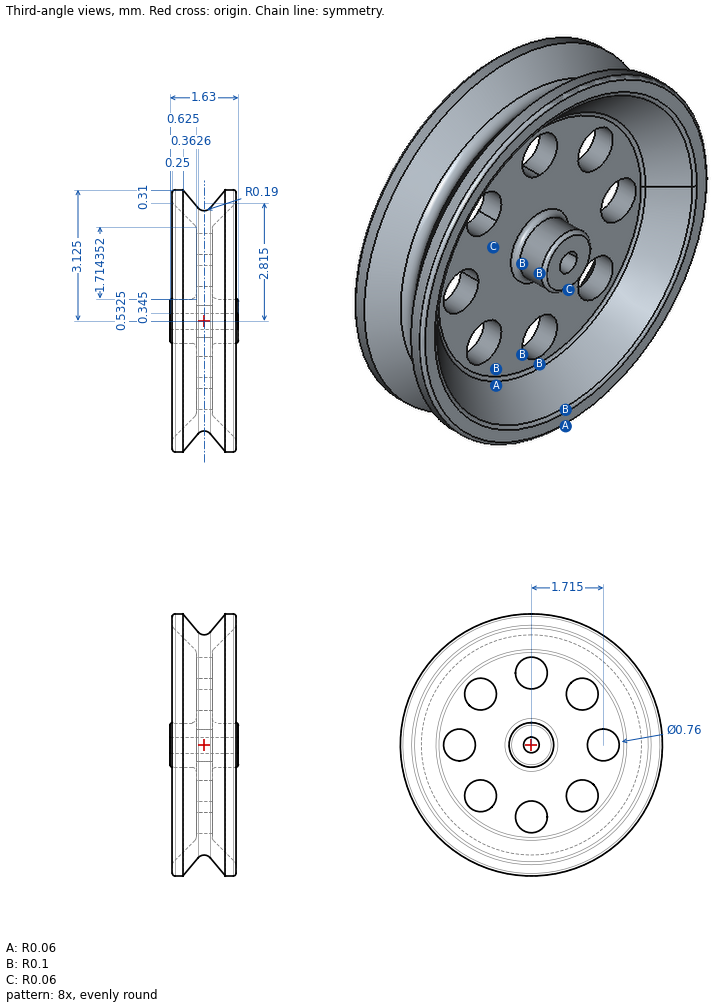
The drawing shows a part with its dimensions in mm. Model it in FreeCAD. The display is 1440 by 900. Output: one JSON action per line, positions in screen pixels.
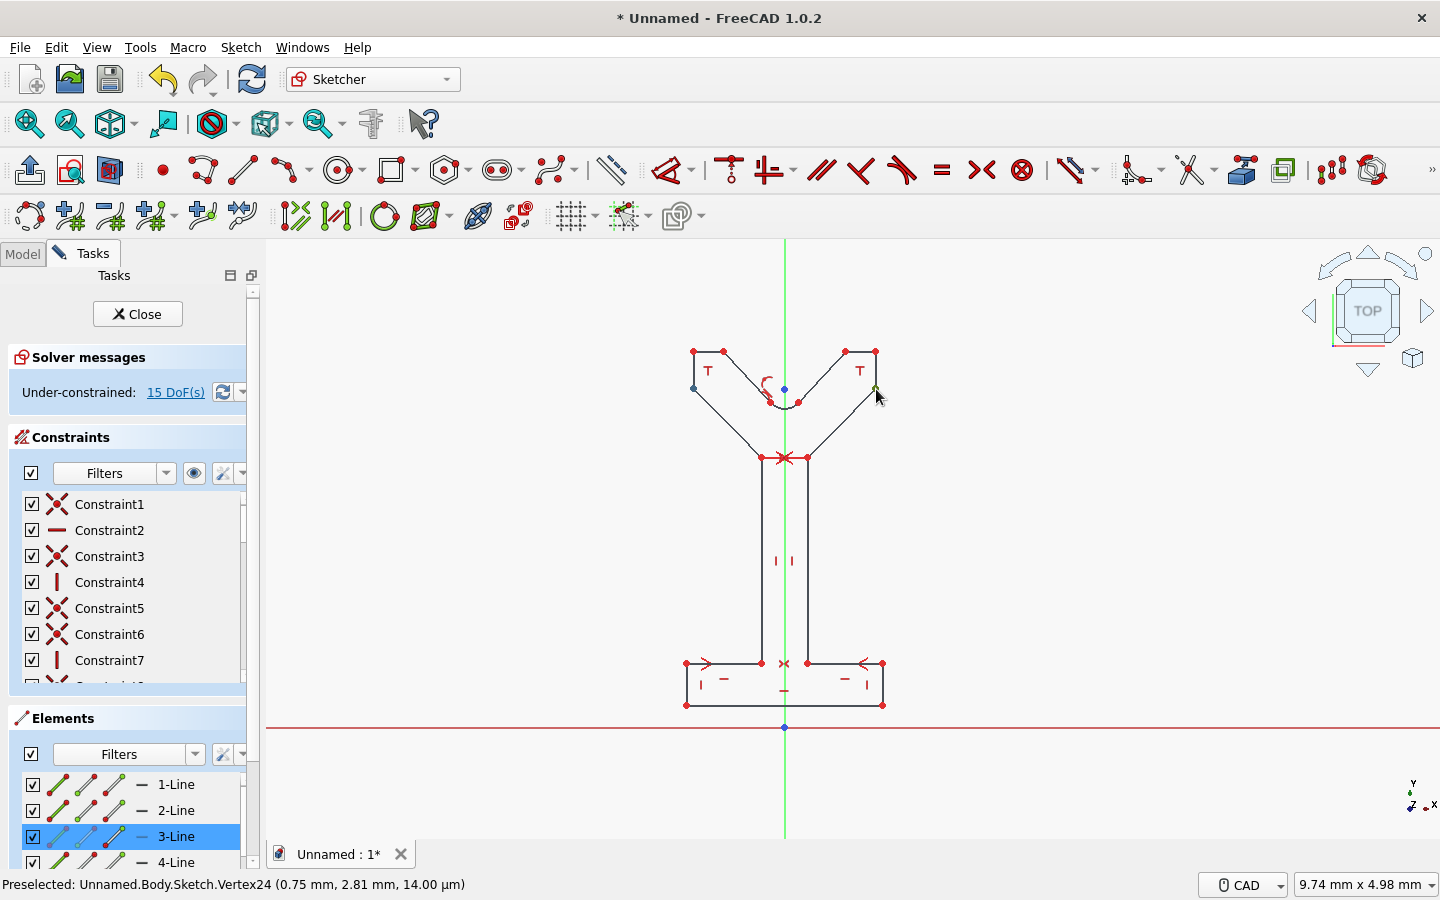
{"action": "left_click", "coordinate": [785, 772]}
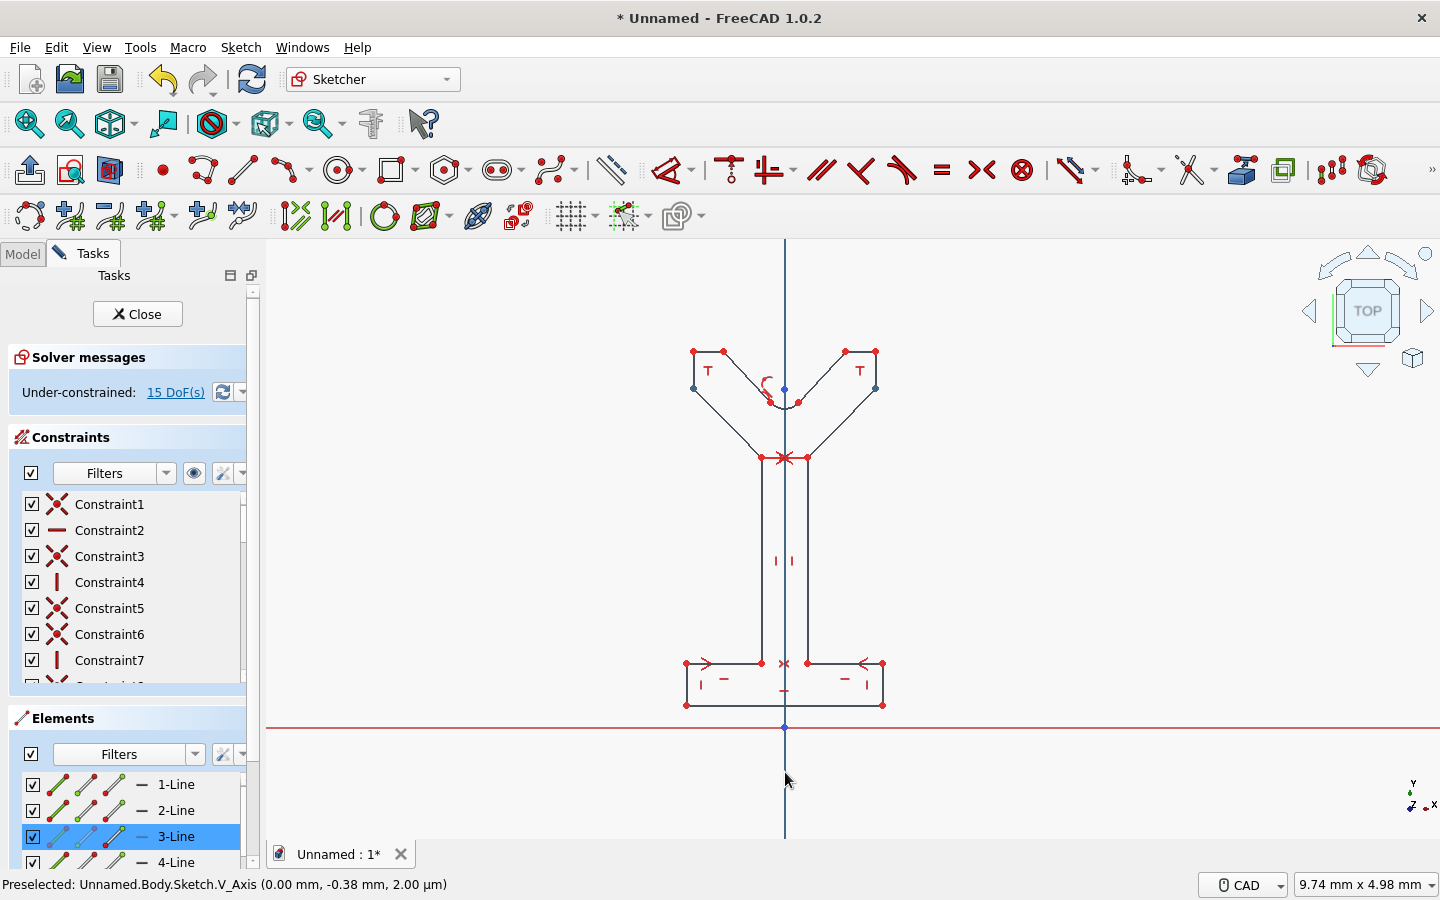
{"action": "left_click", "coordinate": [982, 170]}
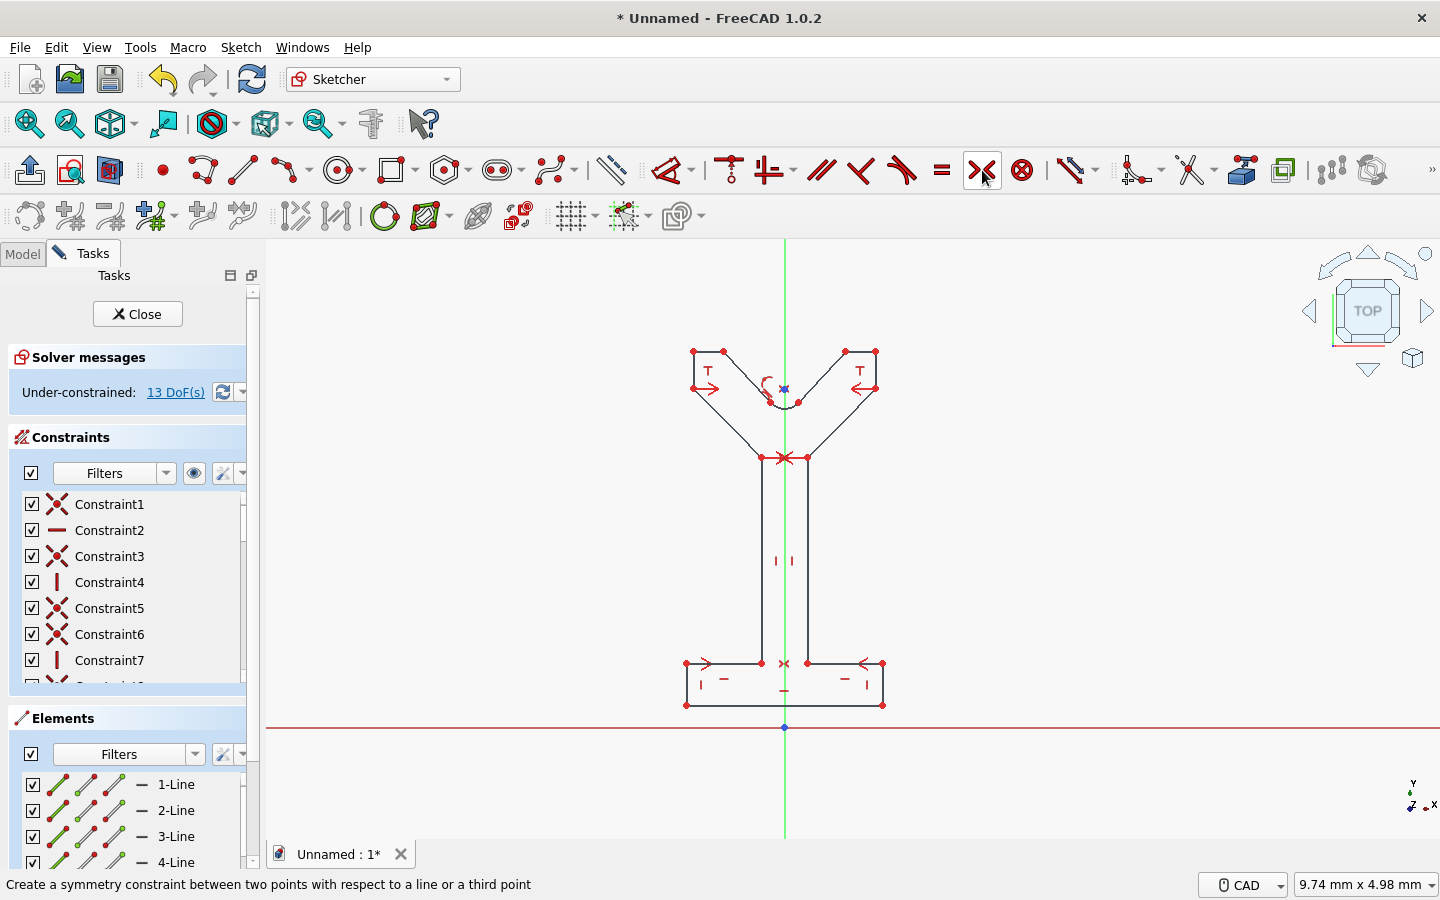
{"action": "left_click", "coordinate": [724, 352]}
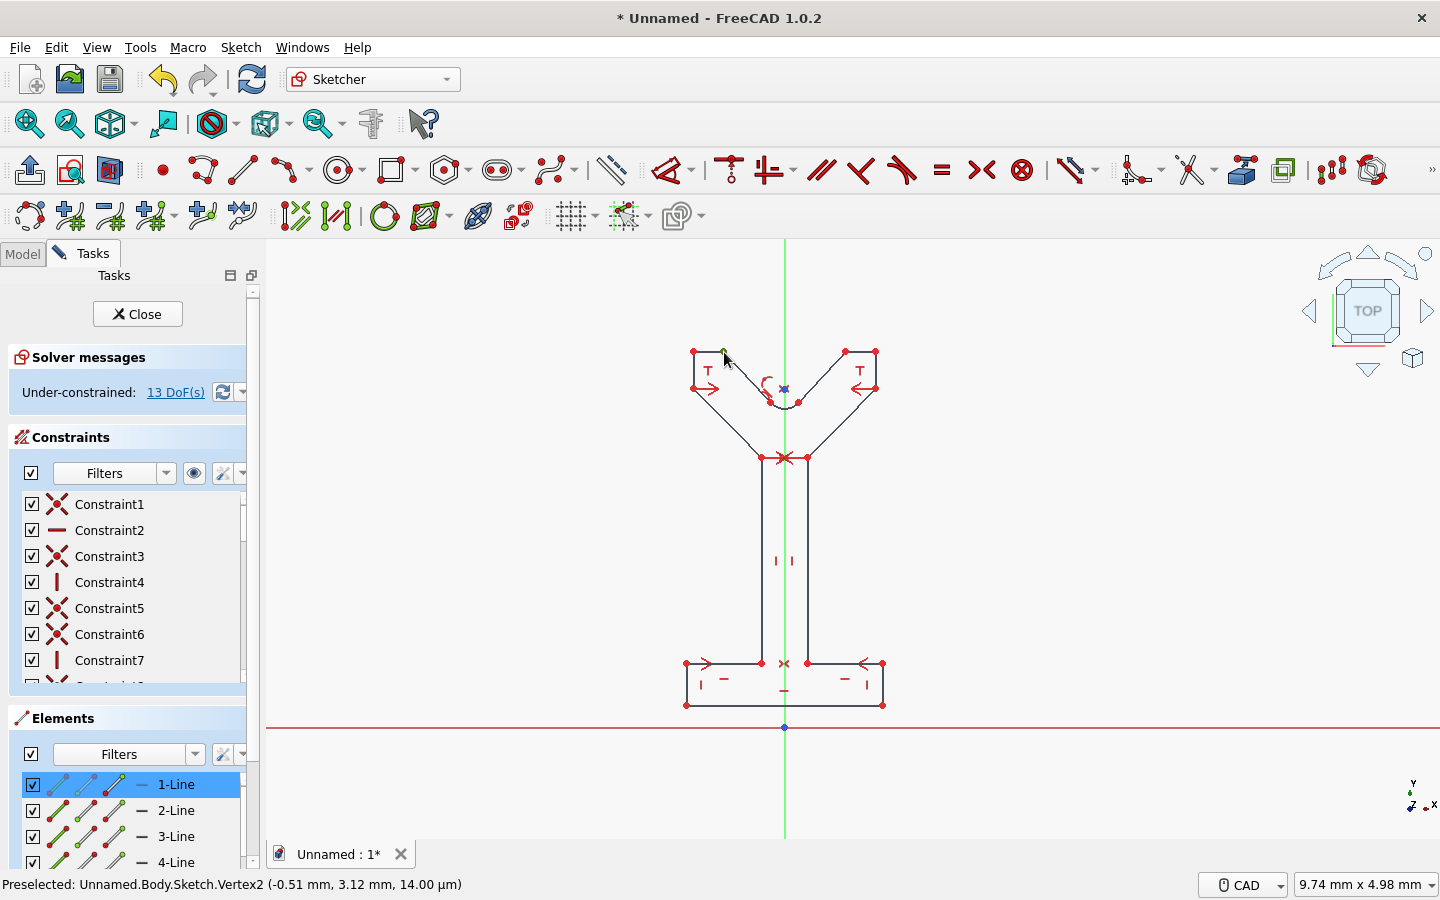
{"action": "left_click", "coordinate": [846, 352]}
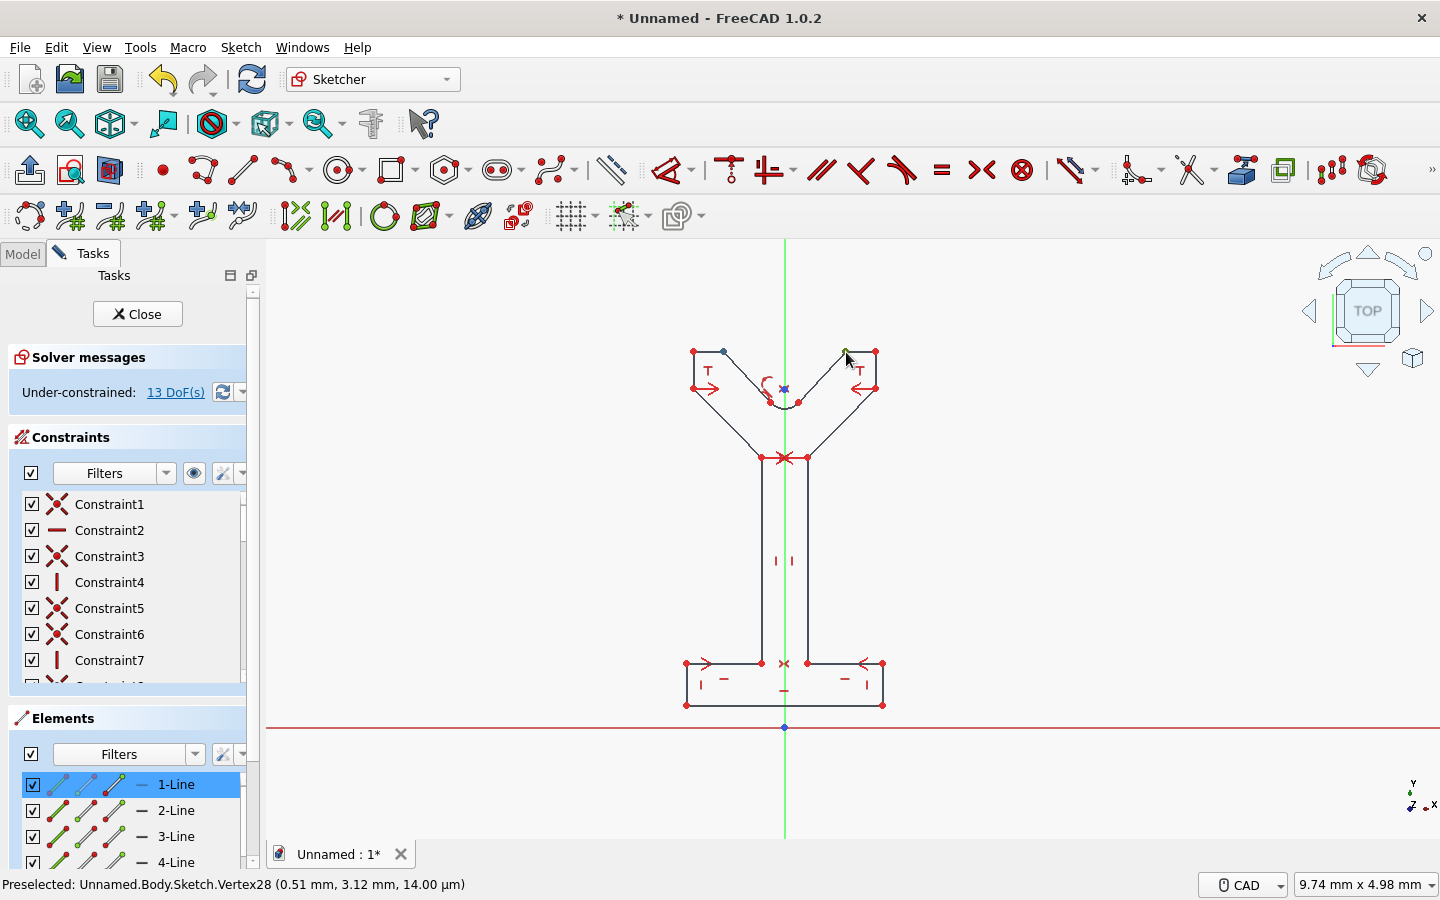
{"action": "left_click", "coordinate": [785, 772]}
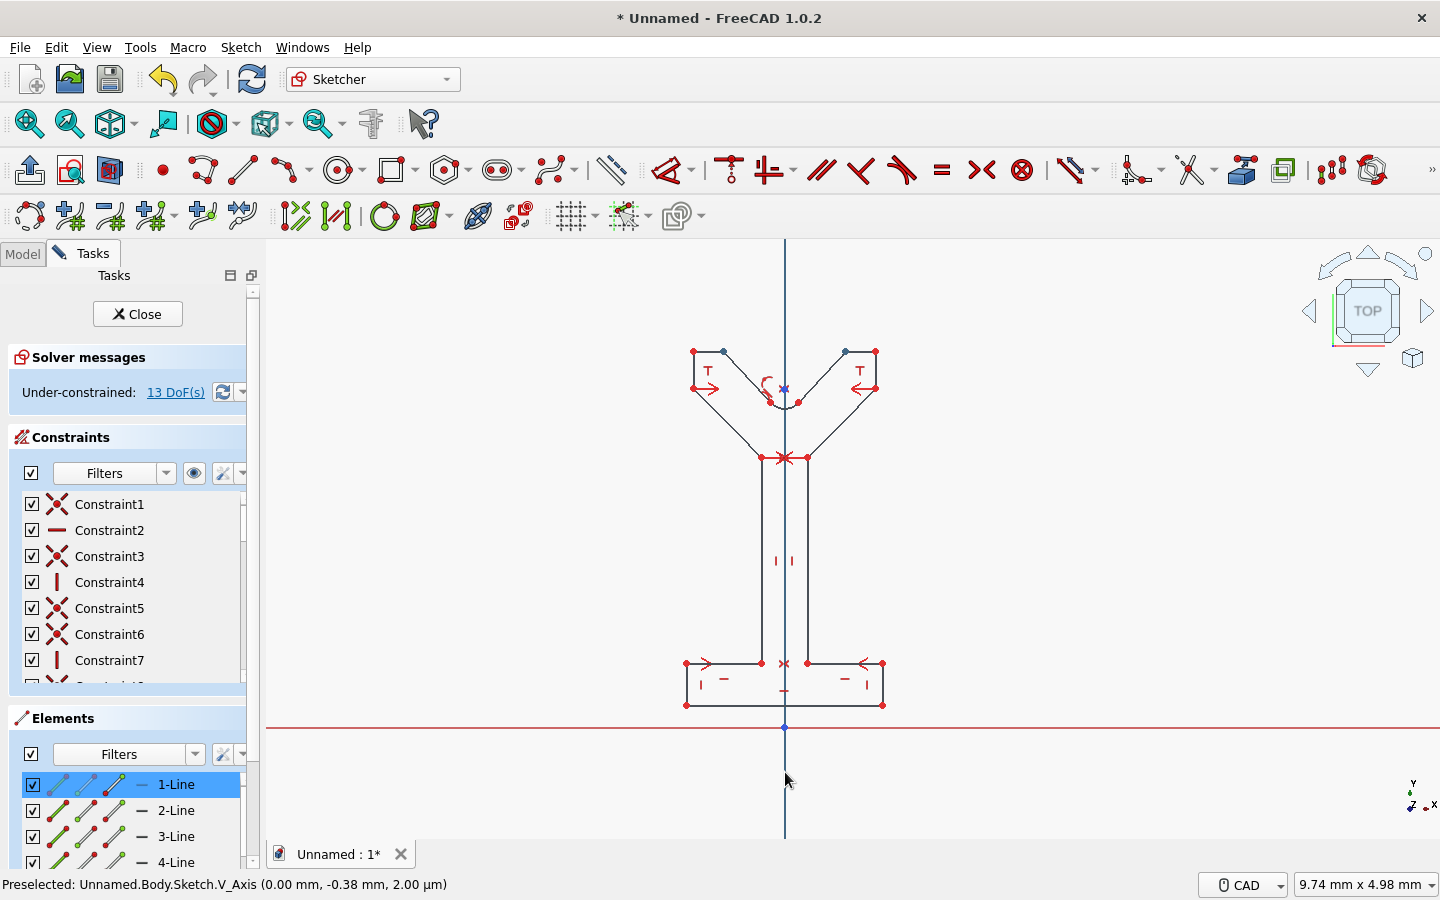
{"action": "left_click", "coordinate": [982, 170]}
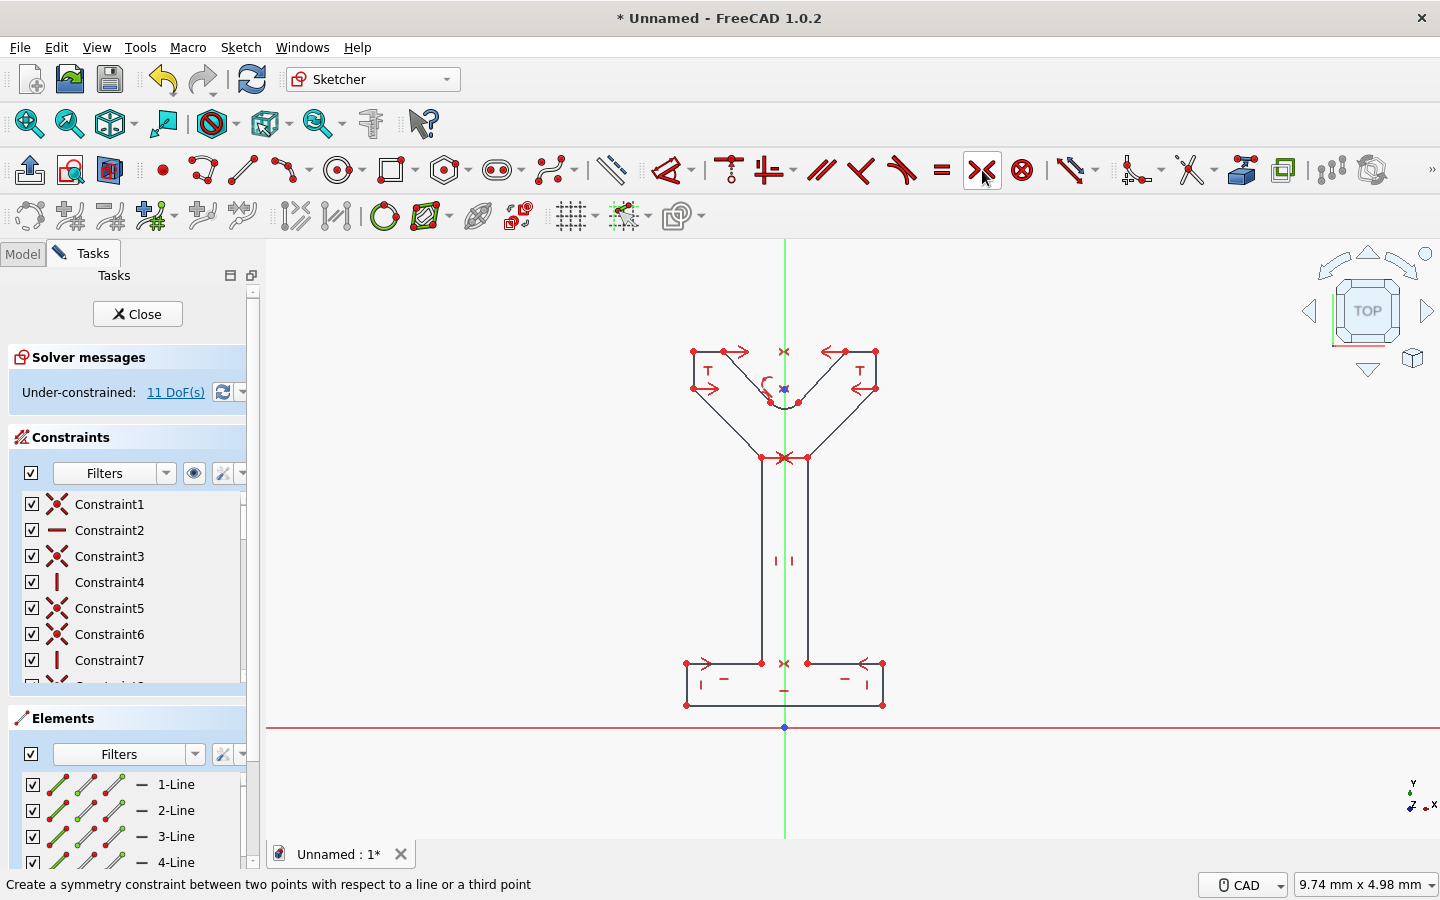
{"action": "key", "text": "d"}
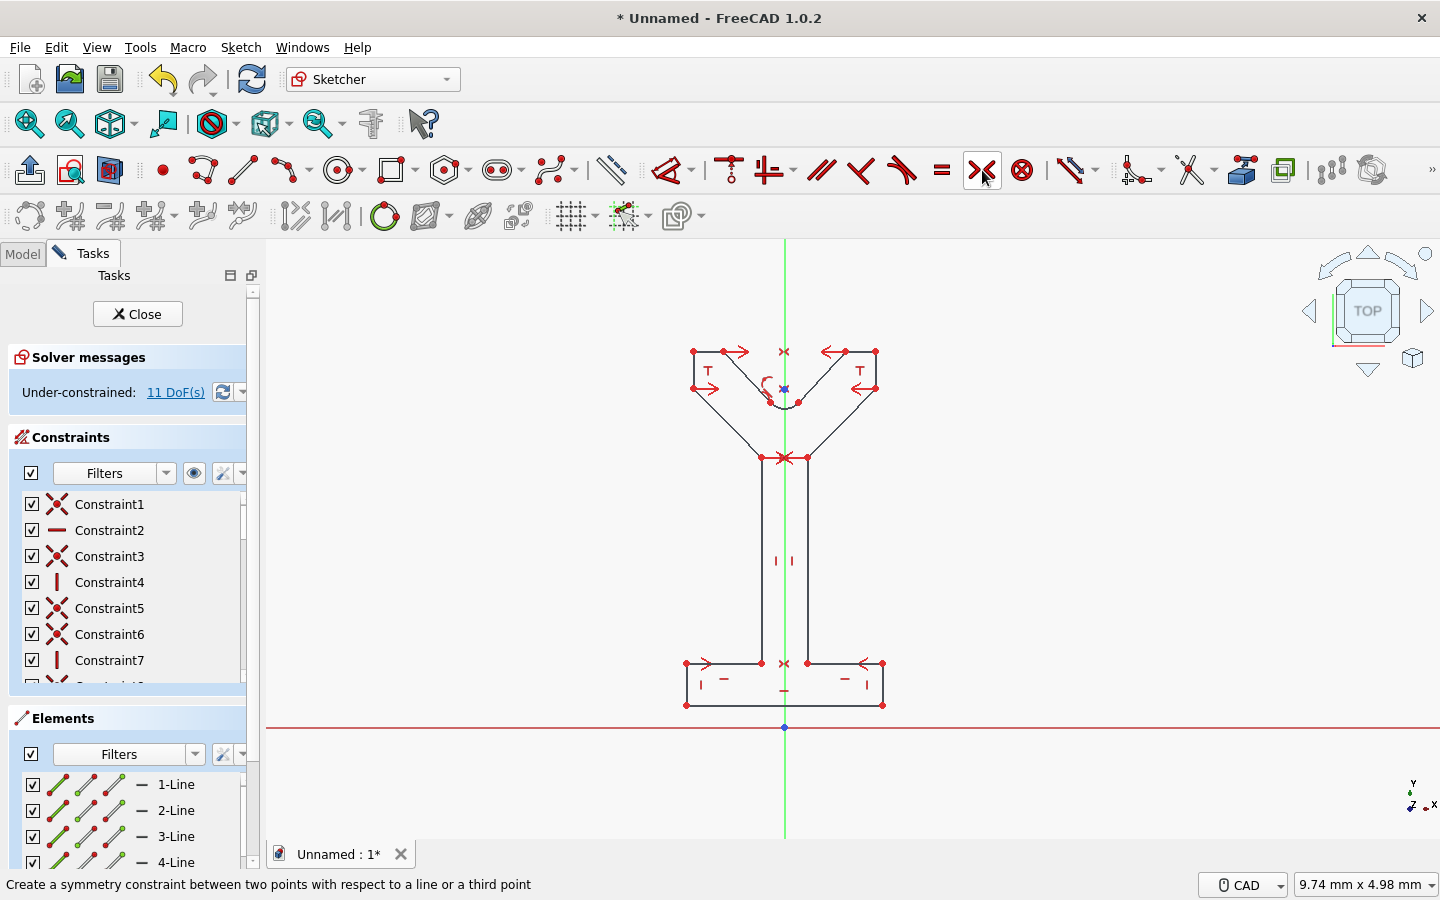
{"action": "scroll", "coordinate": [785, 409], "scroll_direction": "up", "scroll_amount": 3}